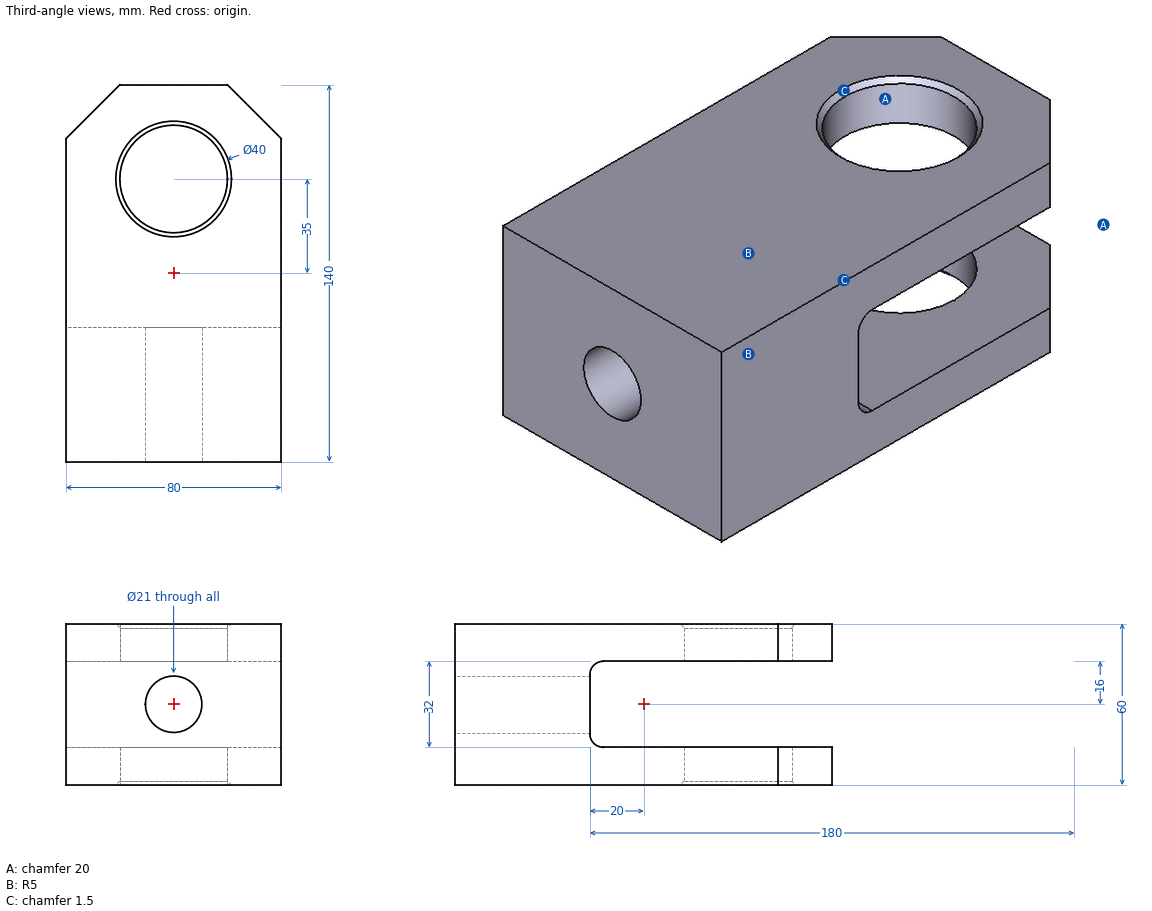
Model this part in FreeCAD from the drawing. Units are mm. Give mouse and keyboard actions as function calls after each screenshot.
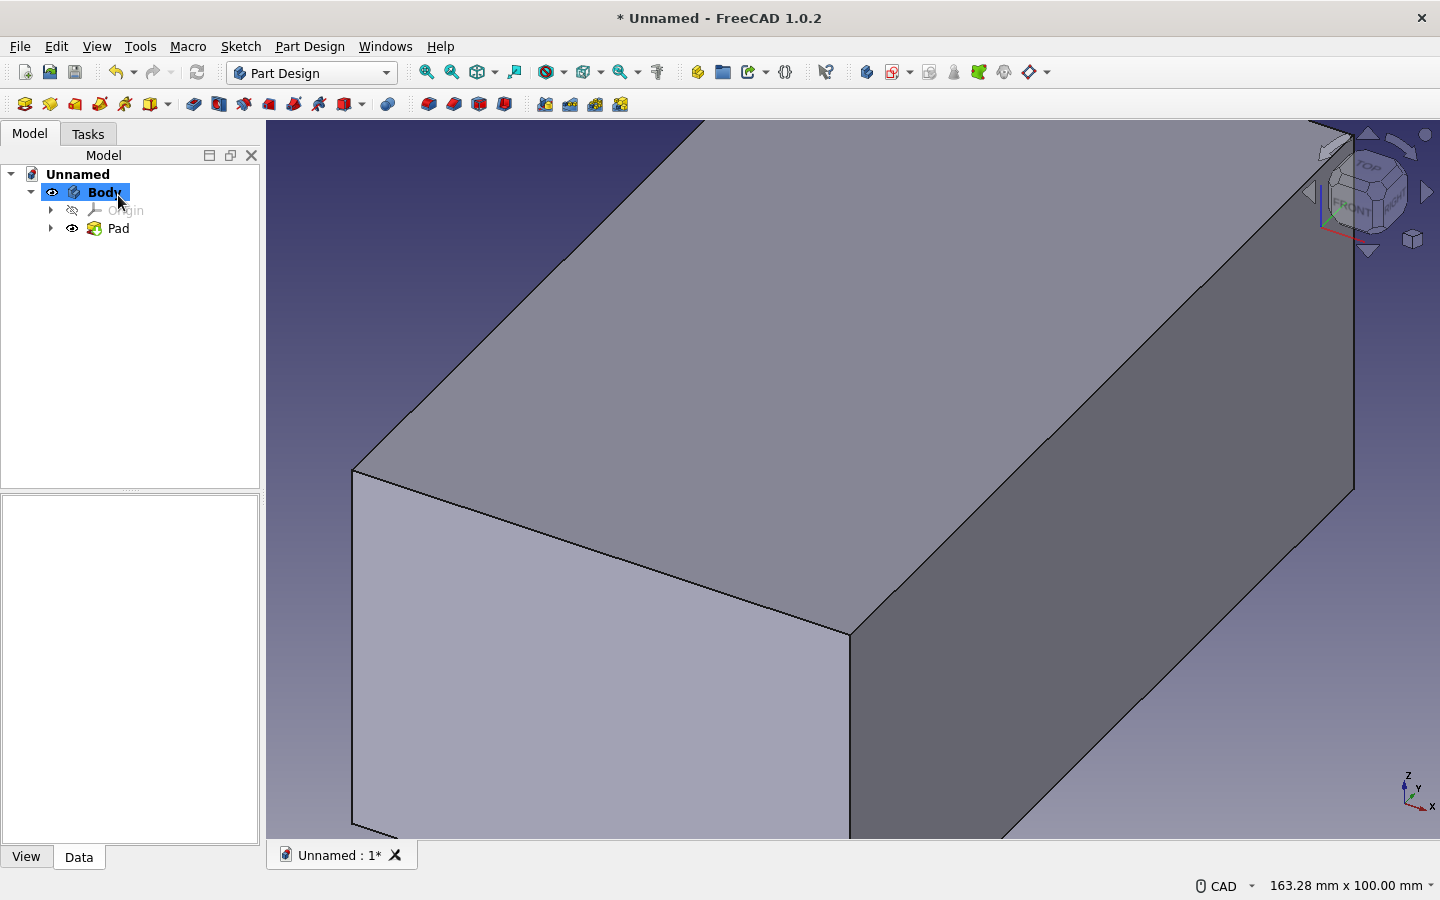
click(427, 72)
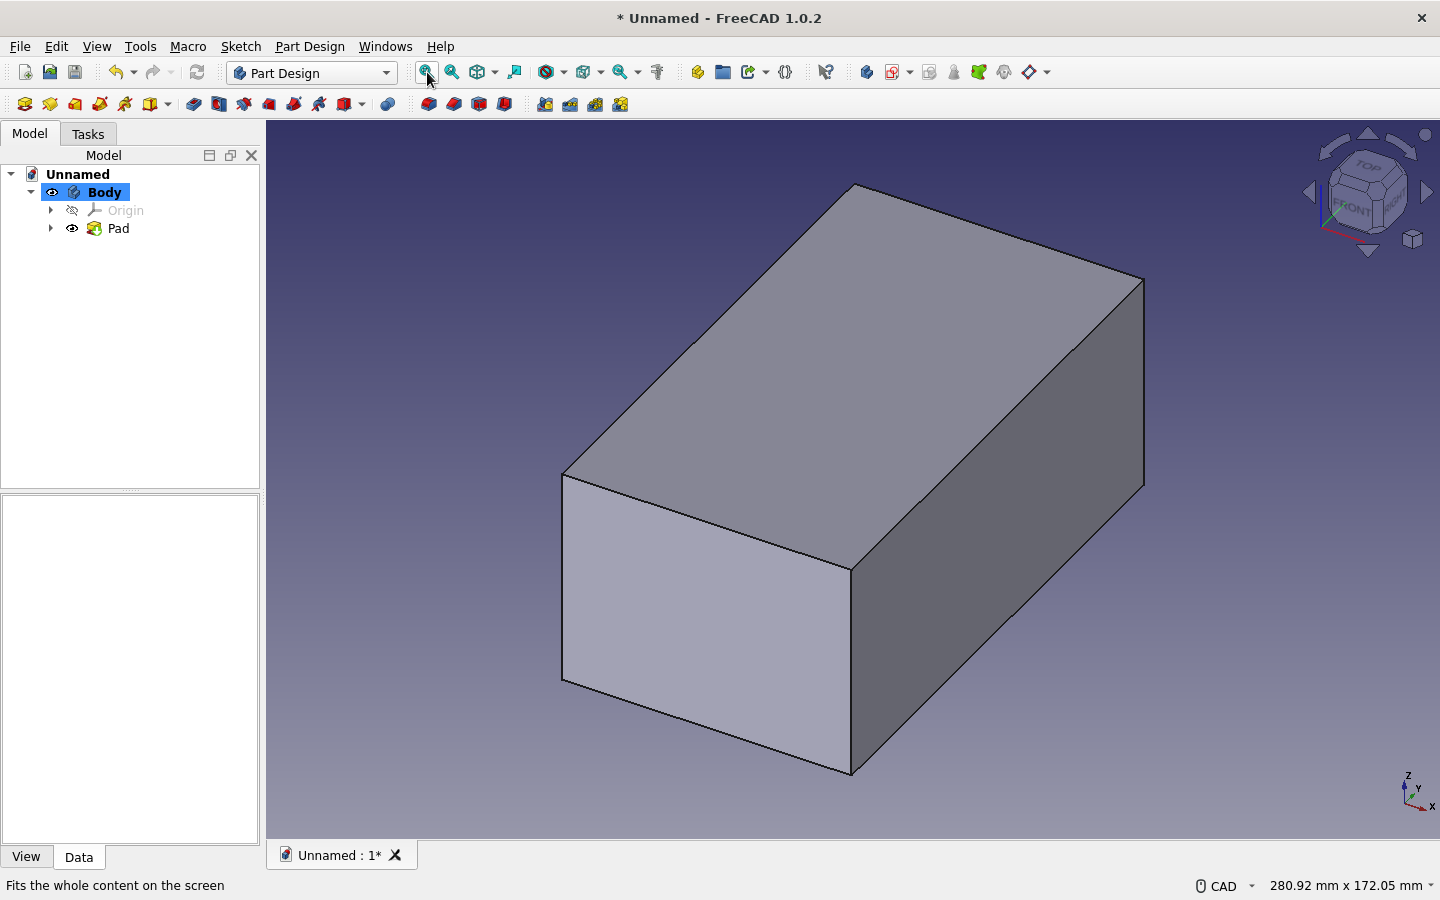
key(0)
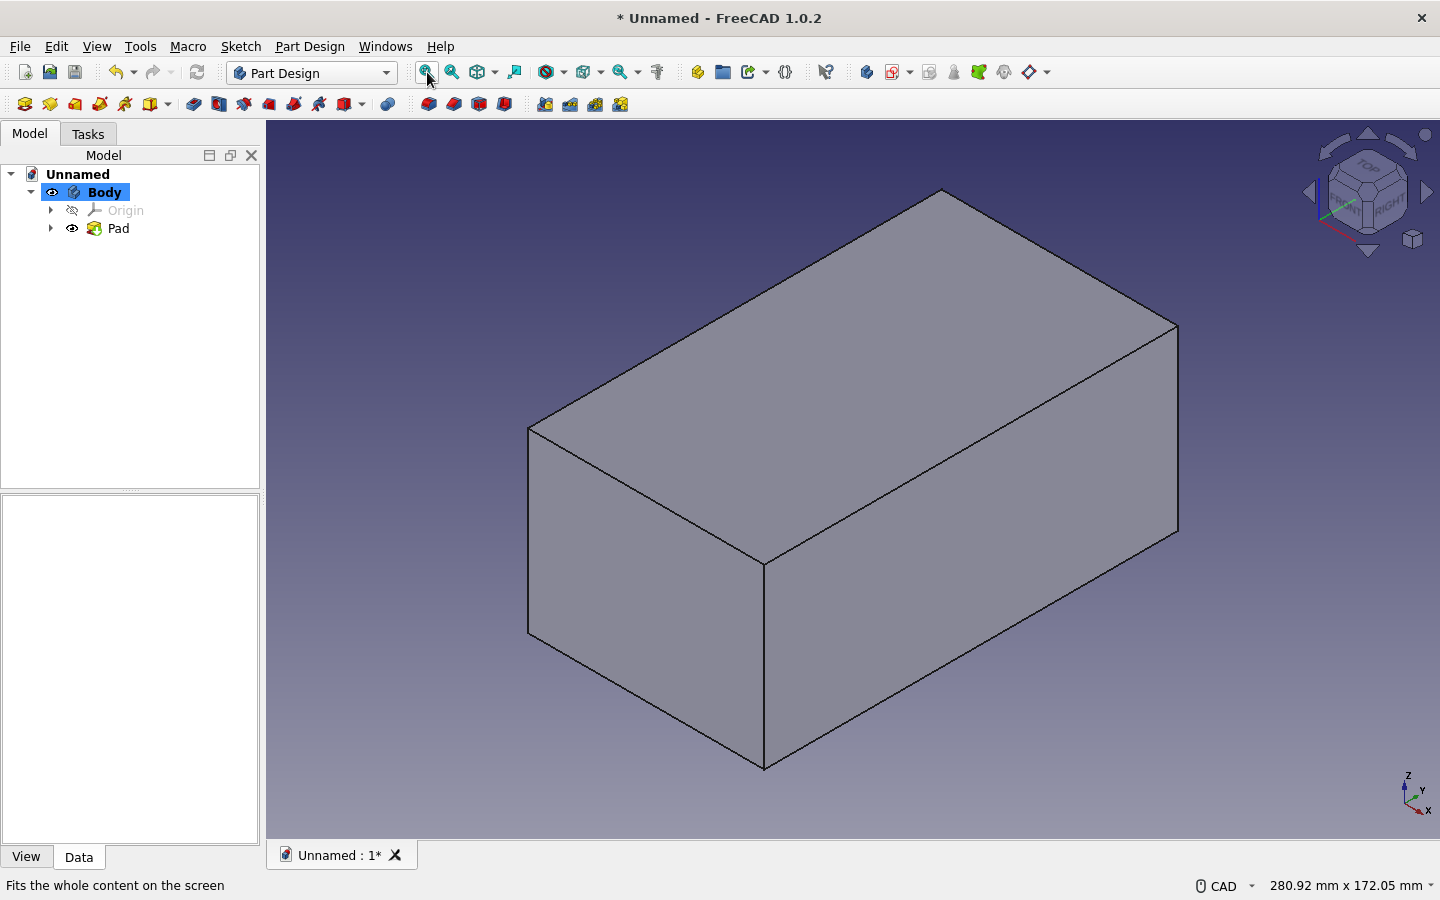
key(2)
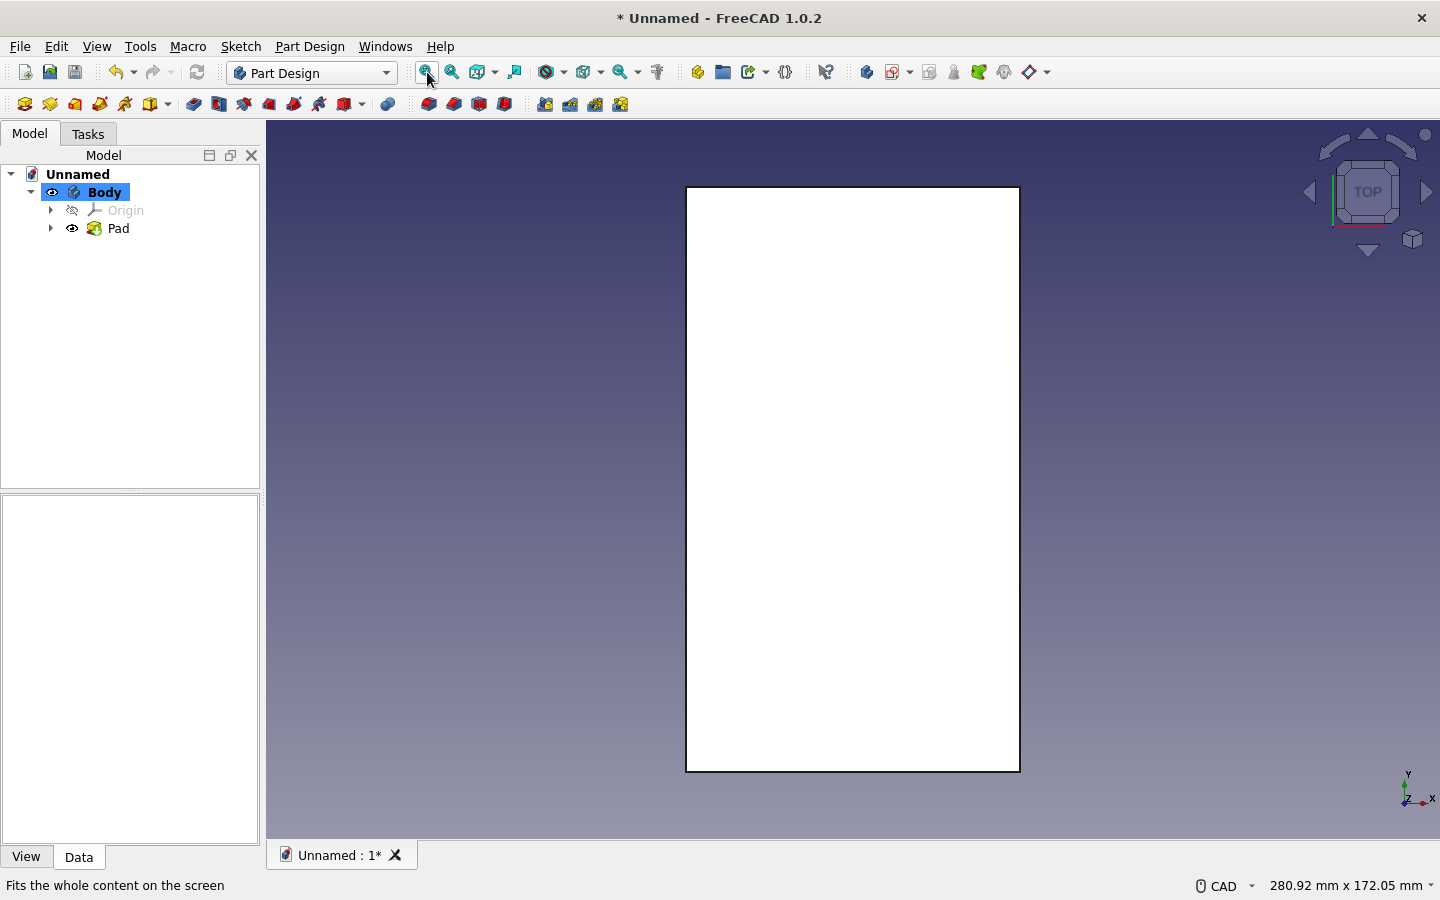
key(1)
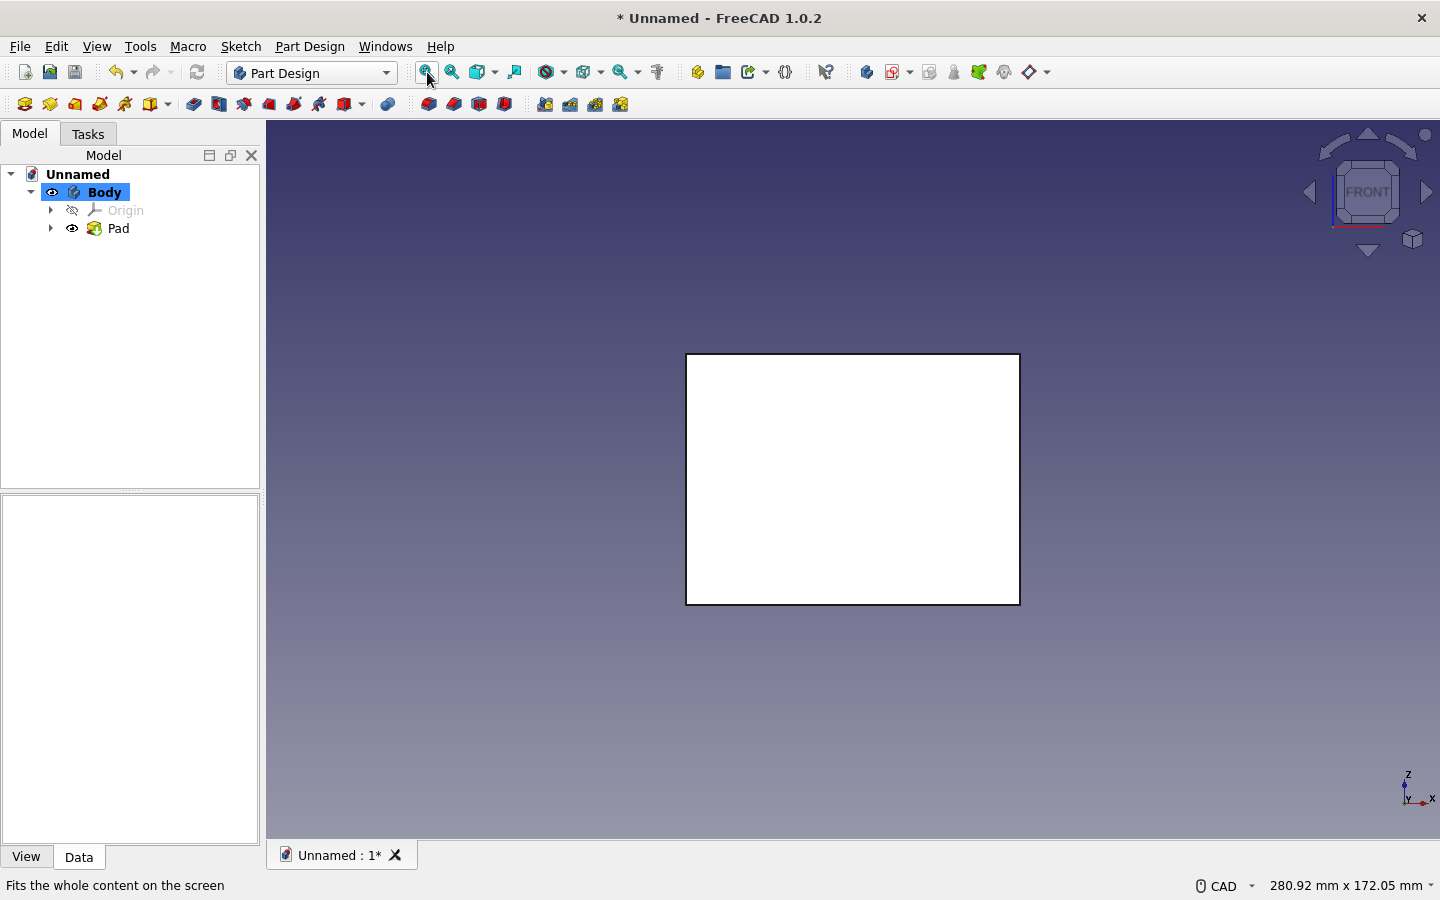
click(427, 72)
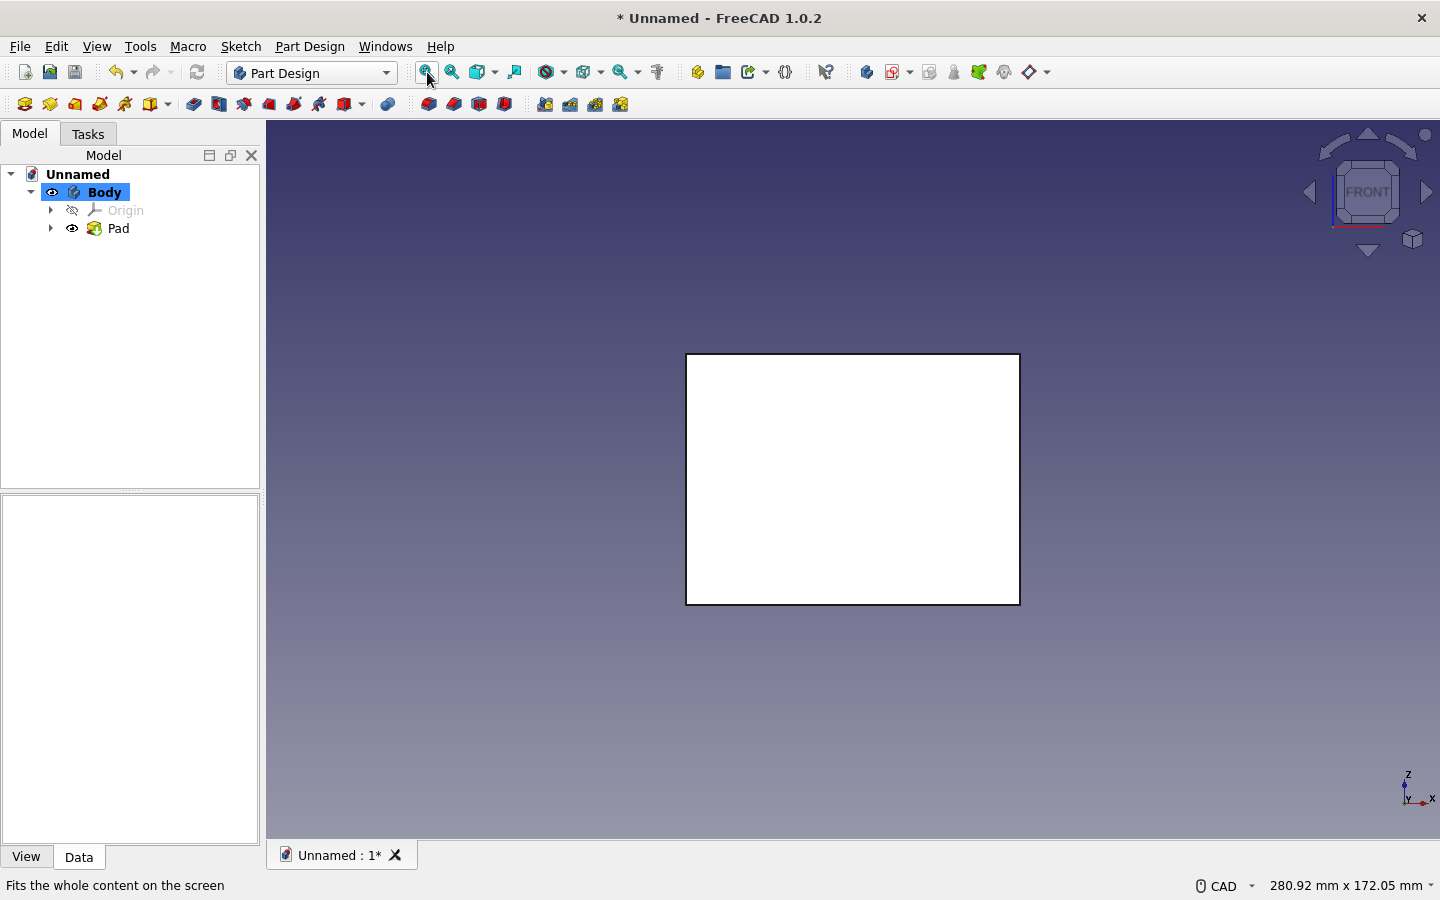
key(3)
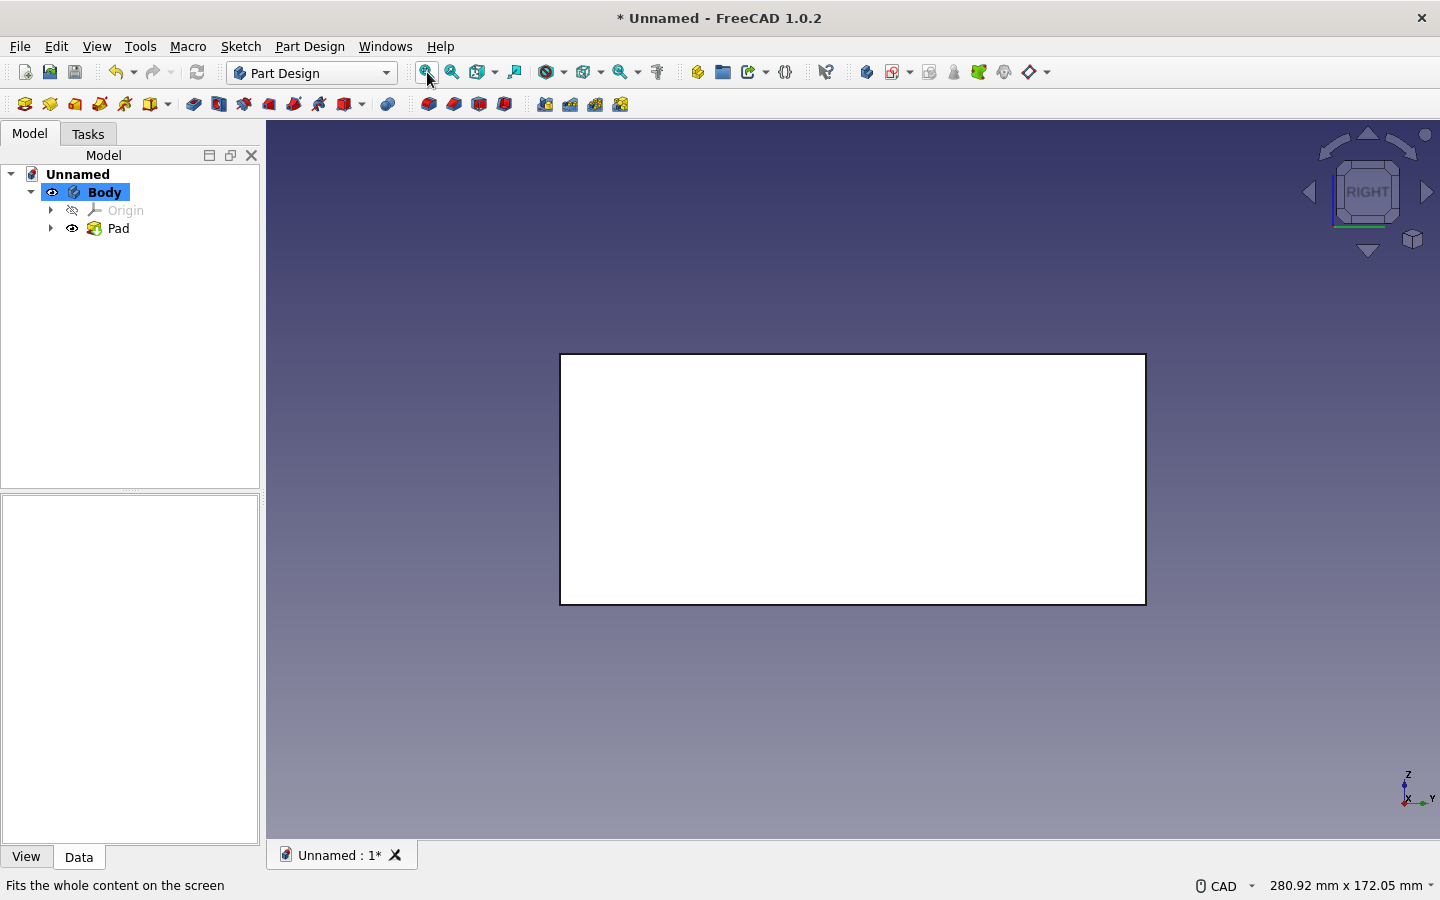
click(1146, 478)